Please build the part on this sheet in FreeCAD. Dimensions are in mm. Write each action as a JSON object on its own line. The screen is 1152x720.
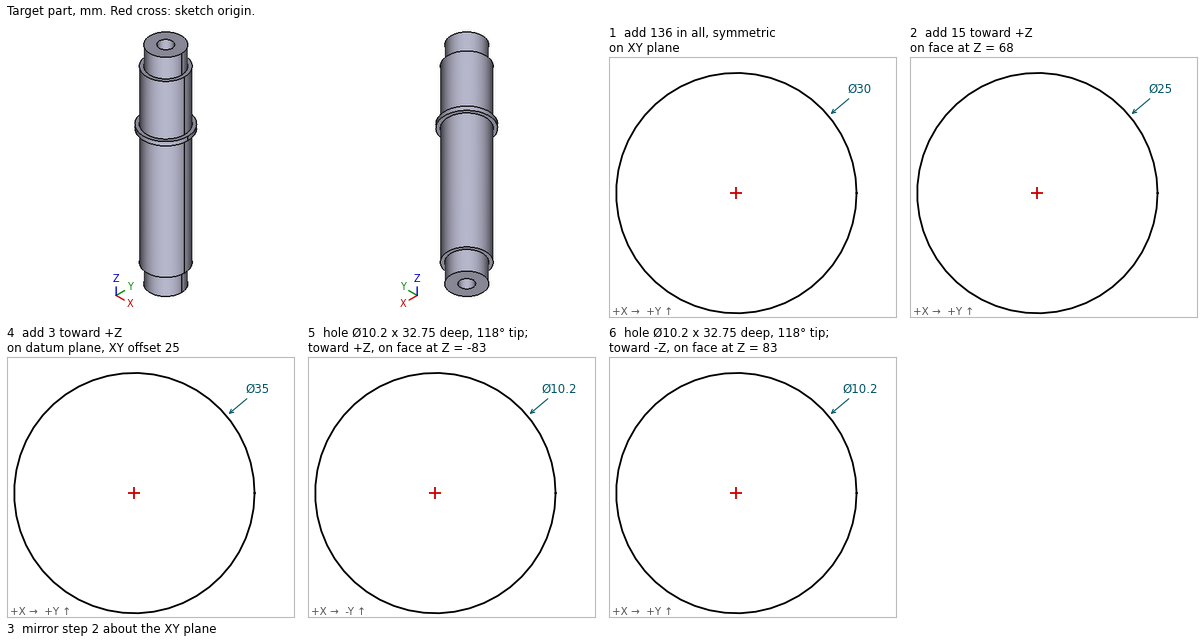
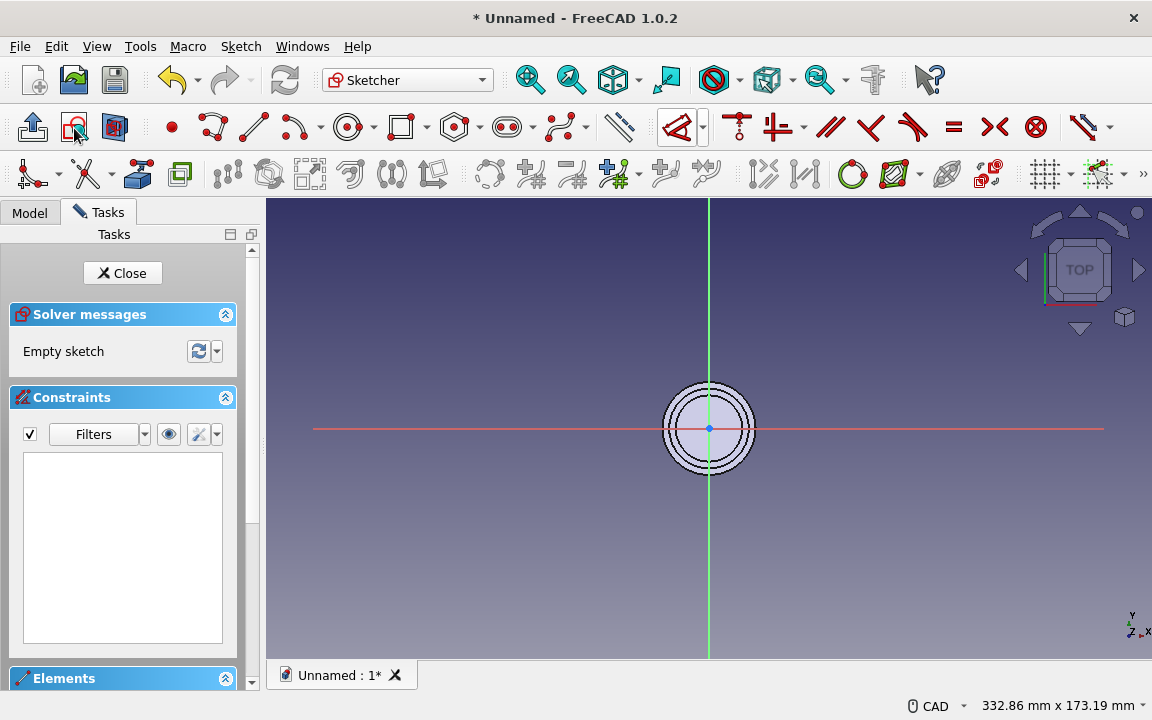
{"action": "scroll", "coordinate": [716, 429], "scroll_direction": "up", "scroll_amount": 12}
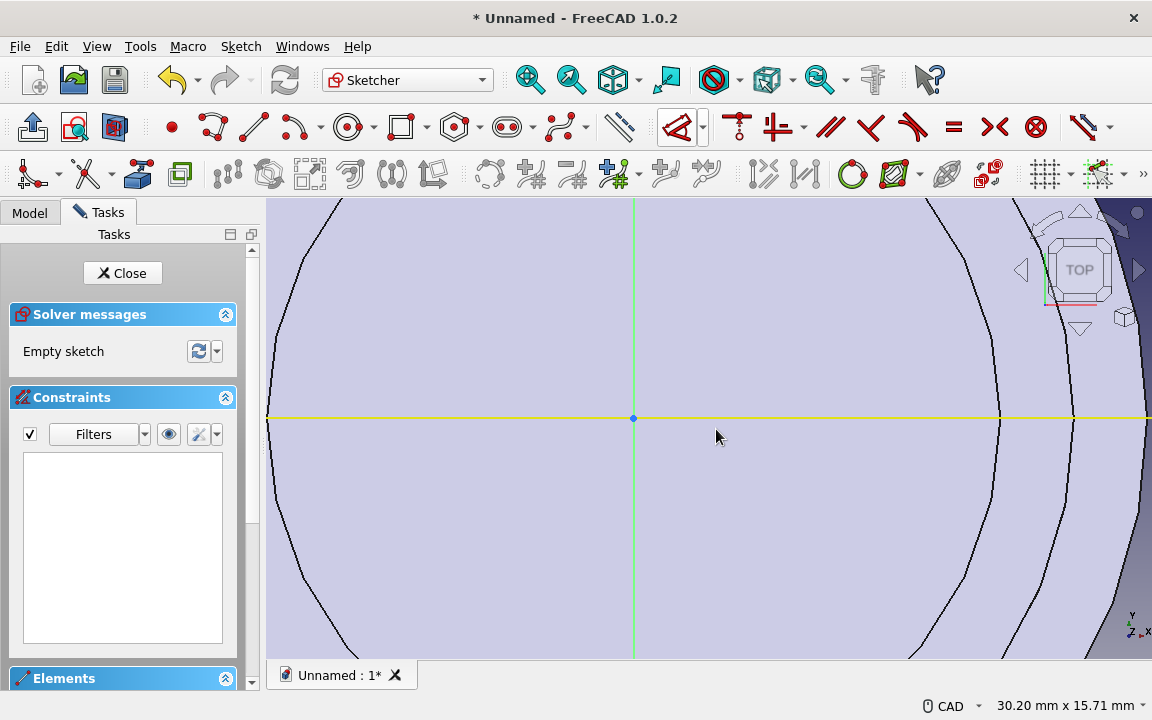
{"action": "left_click", "coordinate": [348, 128]}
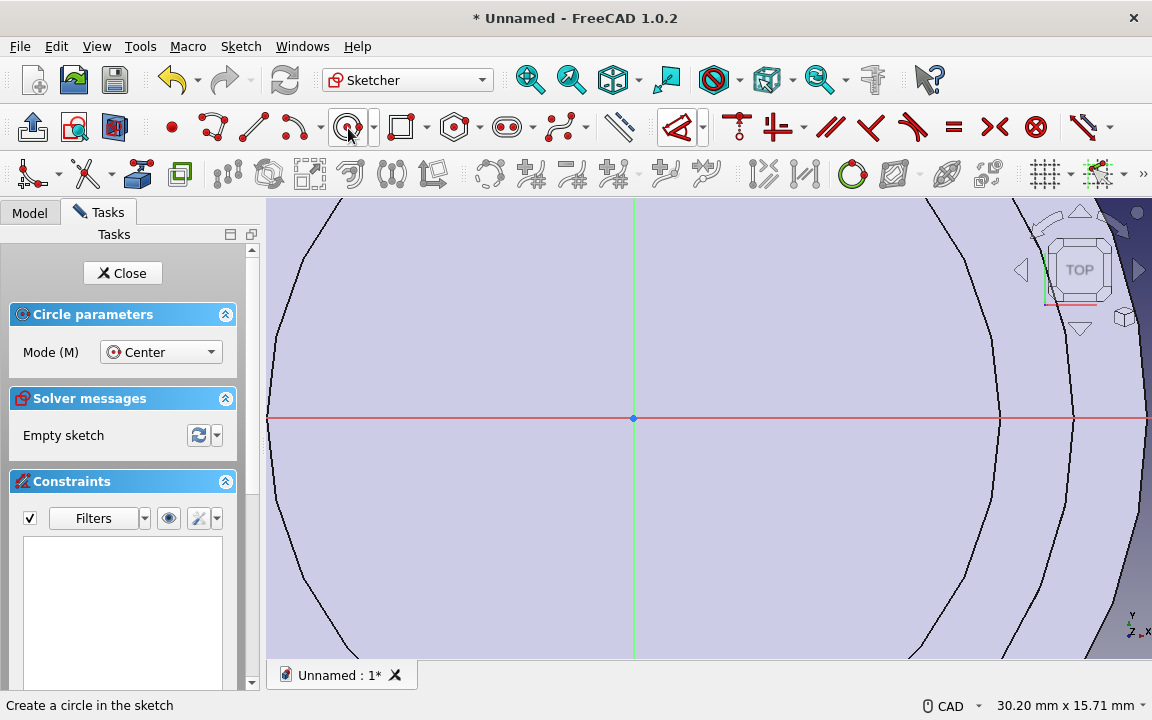
{"action": "left_click", "coordinate": [634, 418]}
{"action": "mouse_move", "coordinate": [740, 313]}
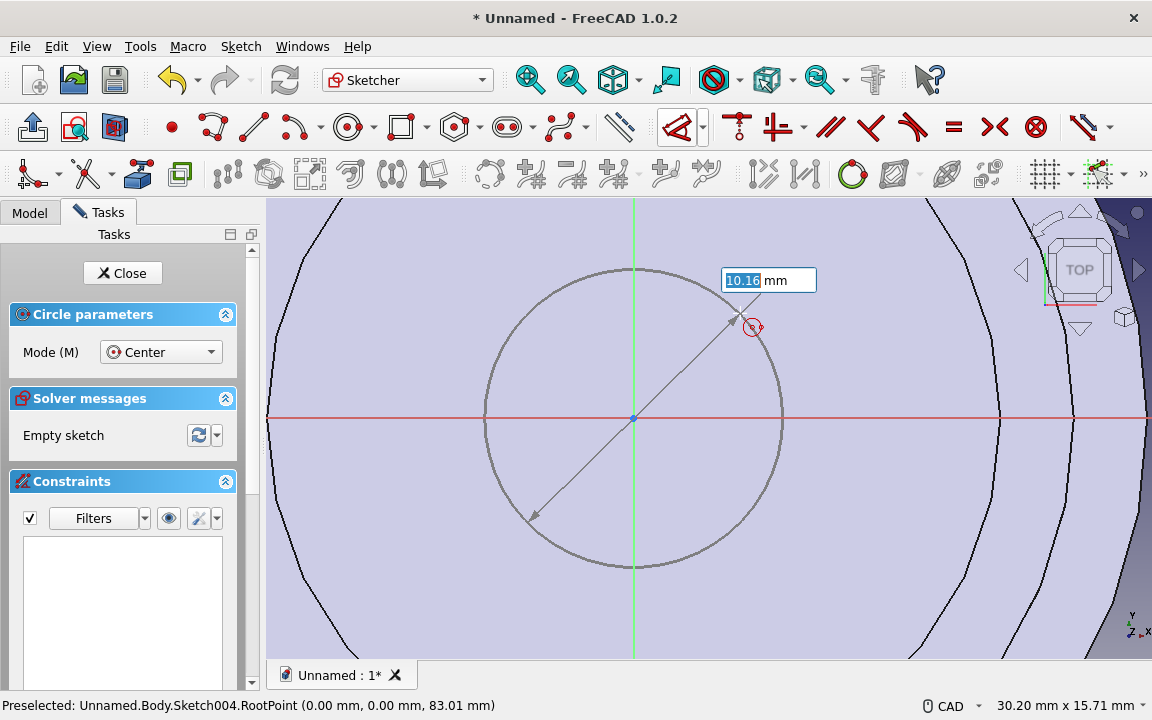
{"action": "type", "text": "10.2"}
{"action": "key", "text": "Return"}
{"action": "key", "text": "Escape"}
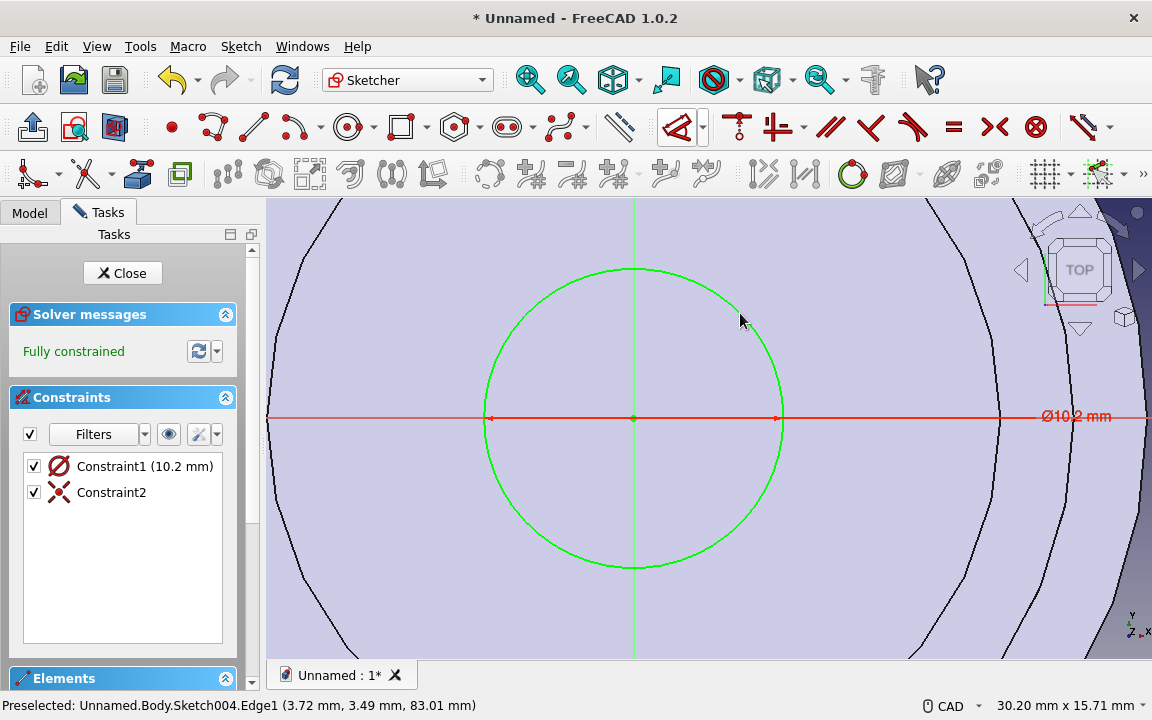
{"action": "left_click", "coordinate": [123, 273]}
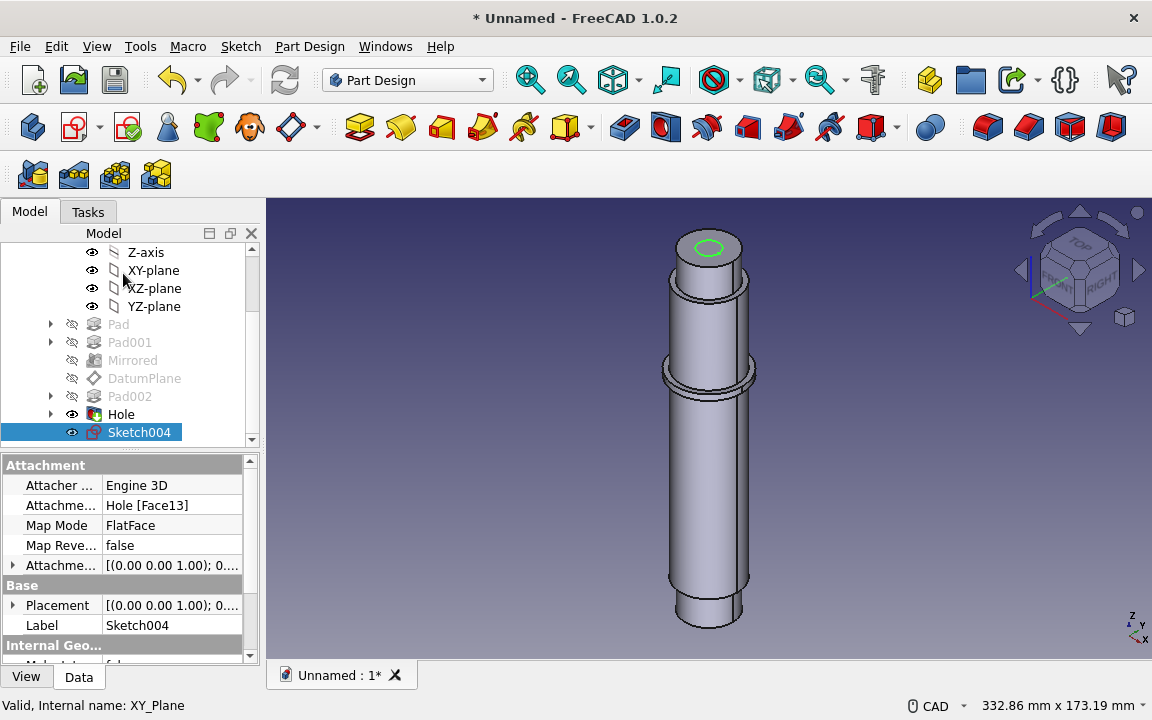
{"action": "left_click", "coordinate": [666, 128]}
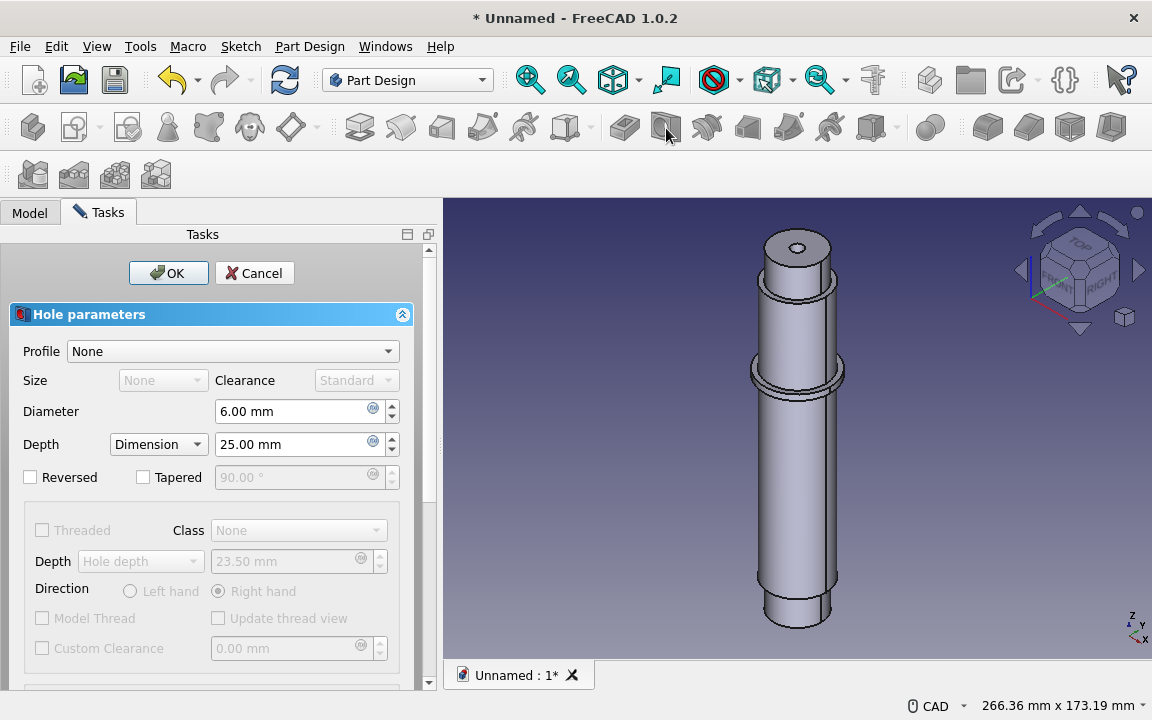
{"action": "triple_click", "coordinate": [300, 412]}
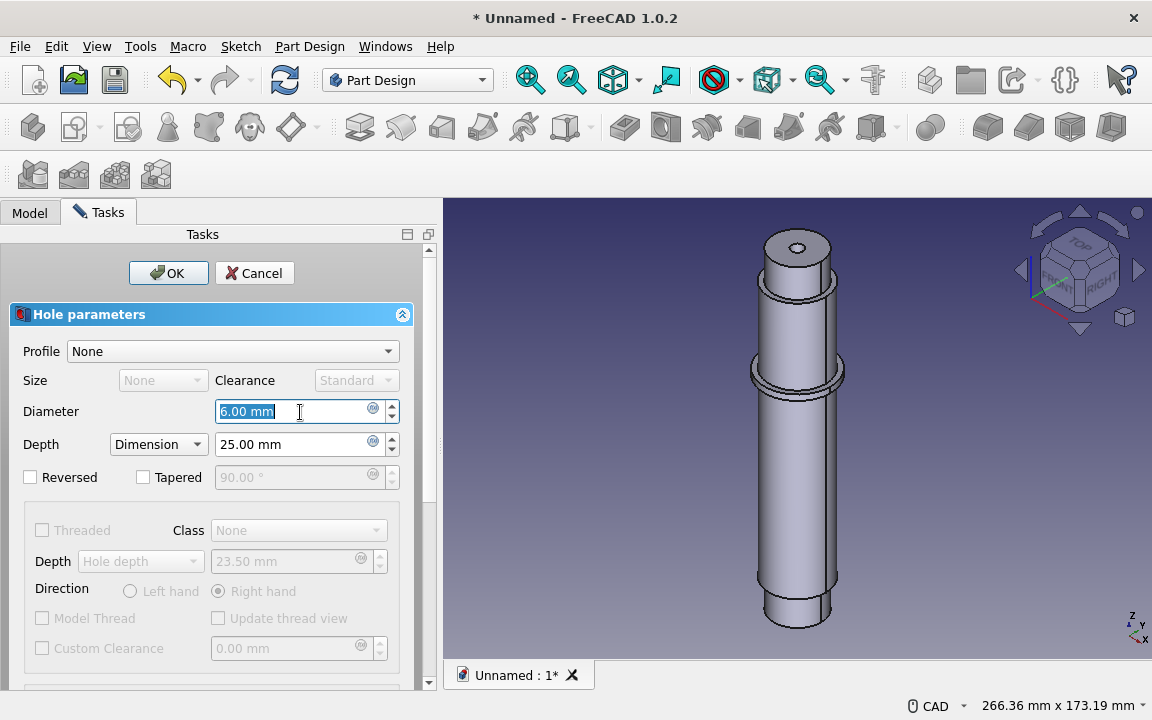
{"action": "type", "text": "10.2"}
{"action": "key", "text": "Tab"}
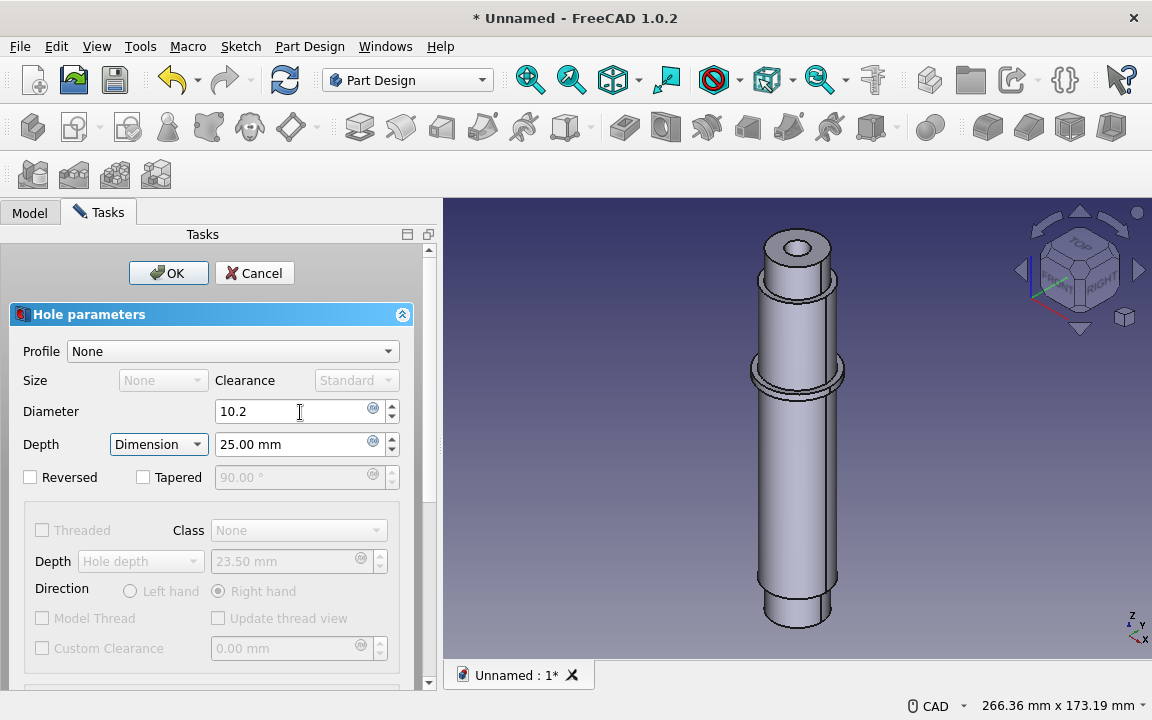
{"action": "triple_click", "coordinate": [300, 444]}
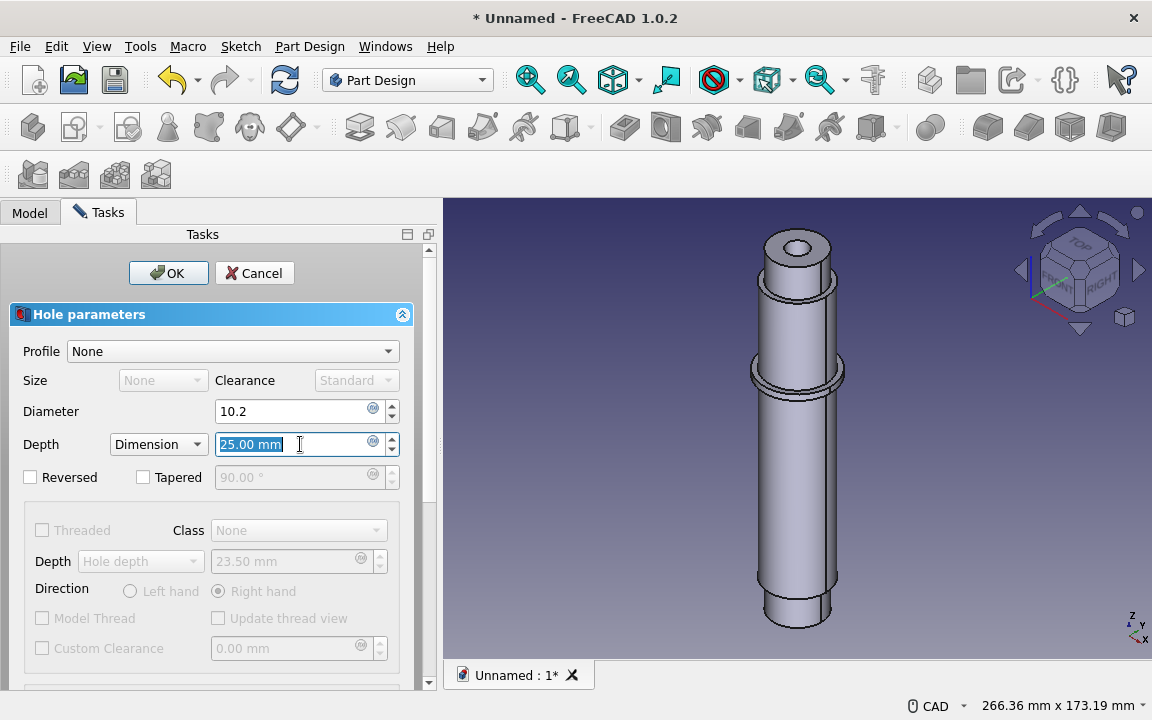
{"action": "type", "text": "32.75"}
{"action": "key", "text": "Tab"}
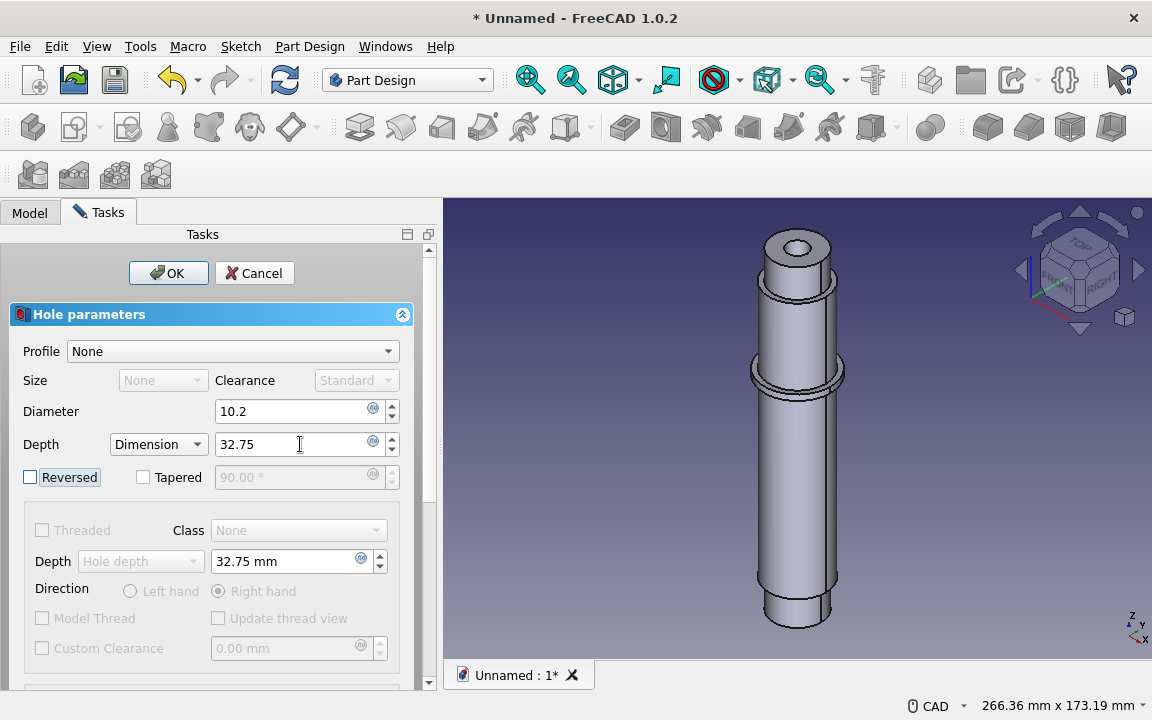
{"action": "left_click", "coordinate": [169, 273]}